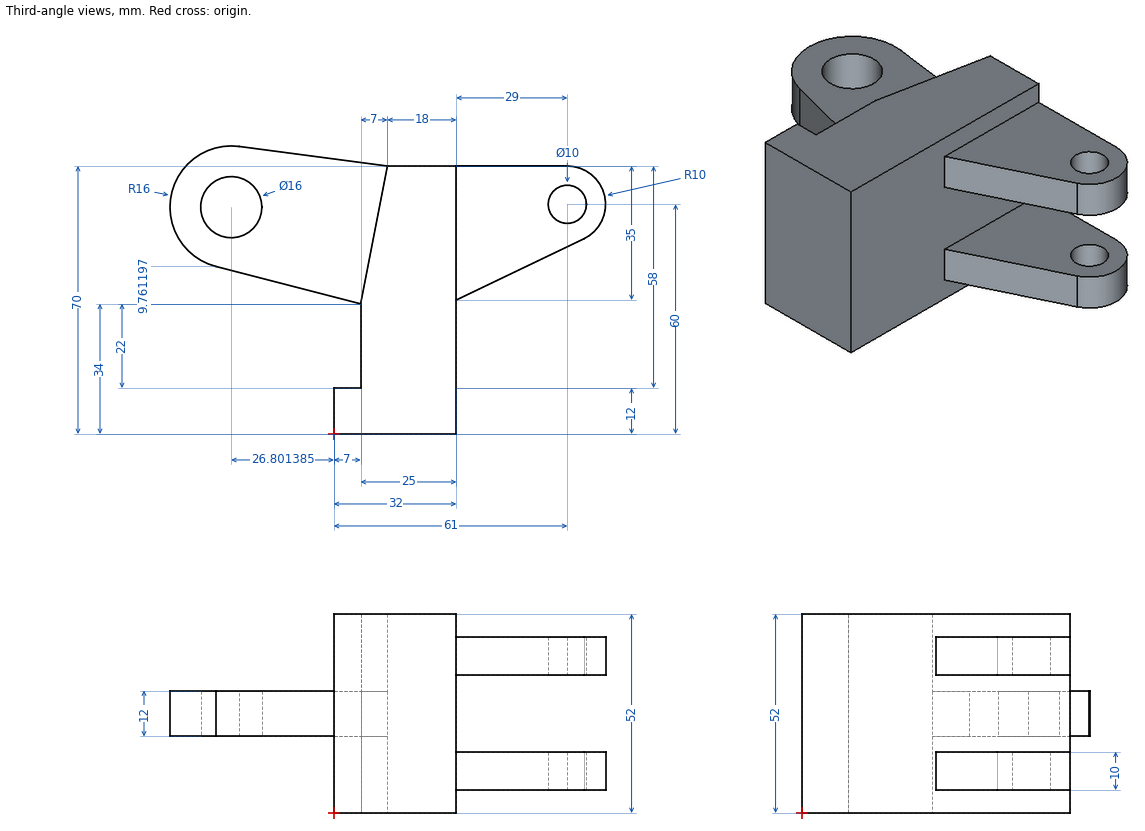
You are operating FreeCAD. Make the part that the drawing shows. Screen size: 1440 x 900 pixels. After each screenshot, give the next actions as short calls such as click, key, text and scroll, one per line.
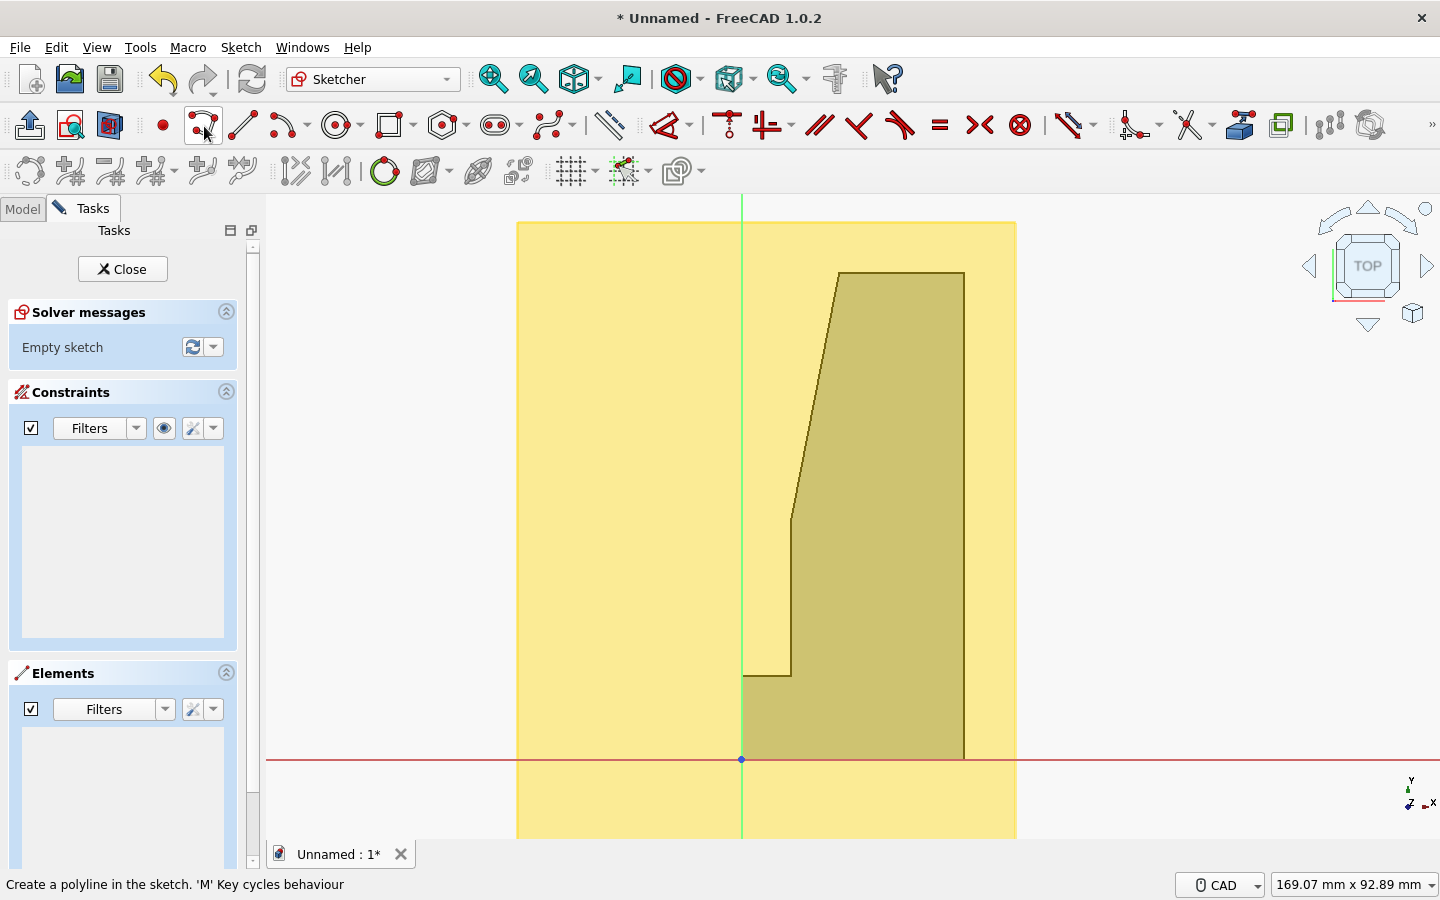
click(1165, 273)
click(964, 273)
click(964, 516)
click(1196, 406)
right_click(1196, 406)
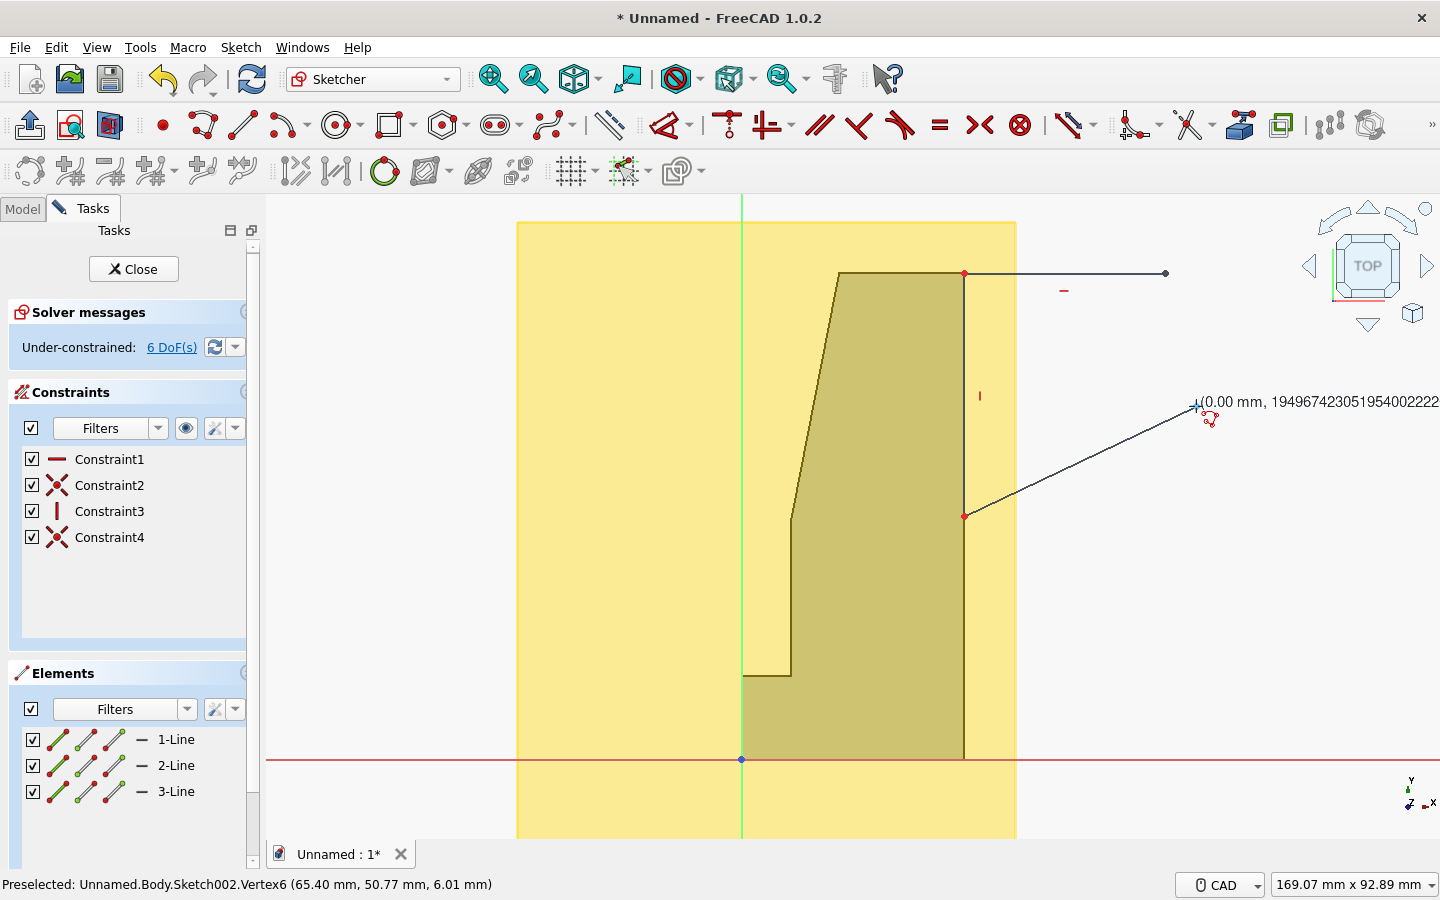
key(g)
key(3)
key(a)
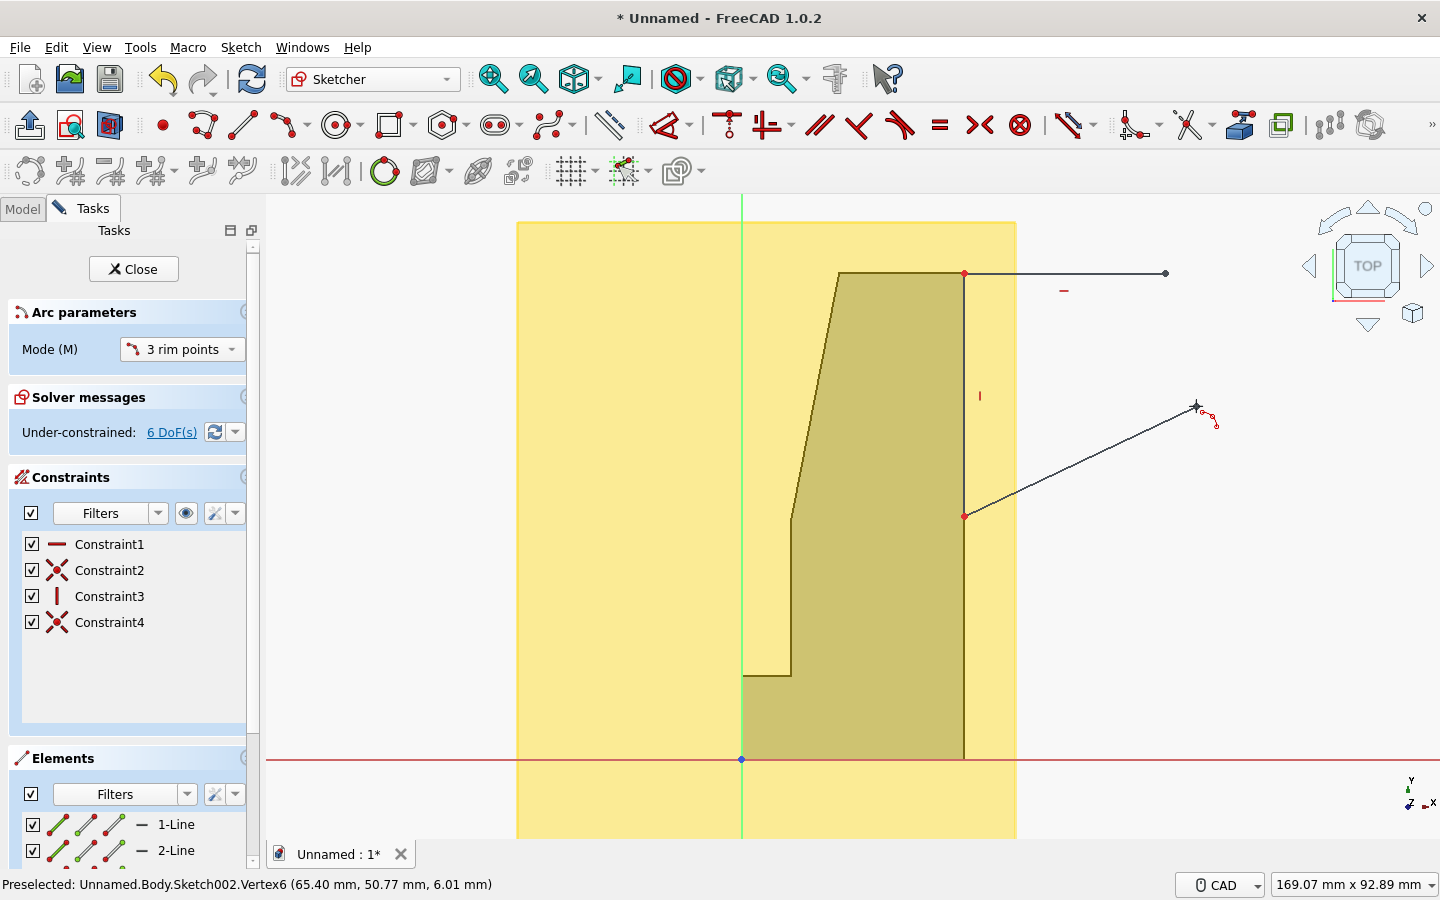
click(1196, 407)
click(1165, 274)
click(1233, 328)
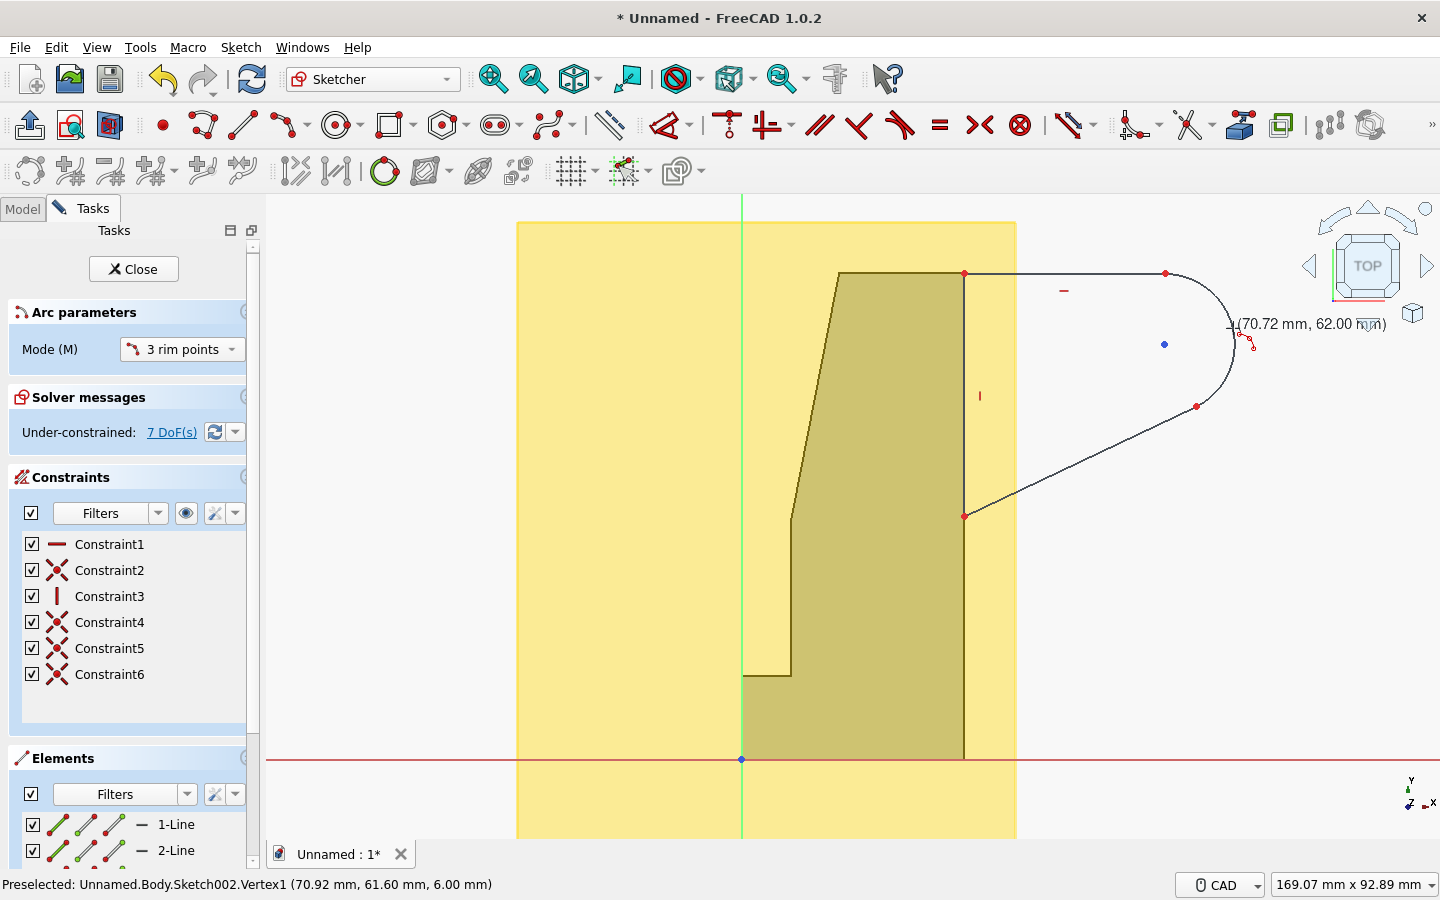
click(336, 126)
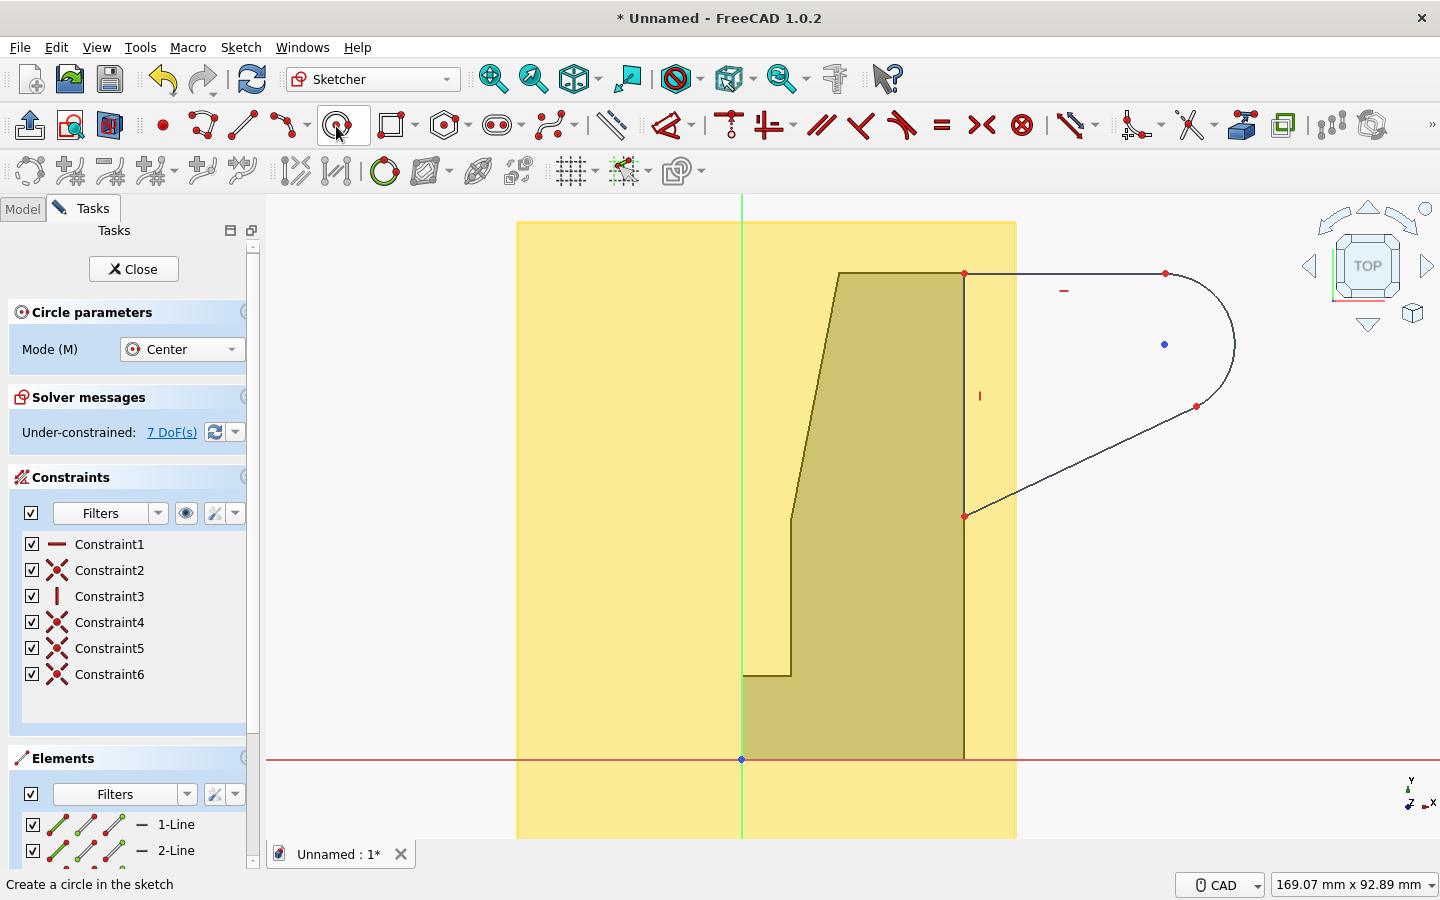
click(1165, 343)
move(1190, 318)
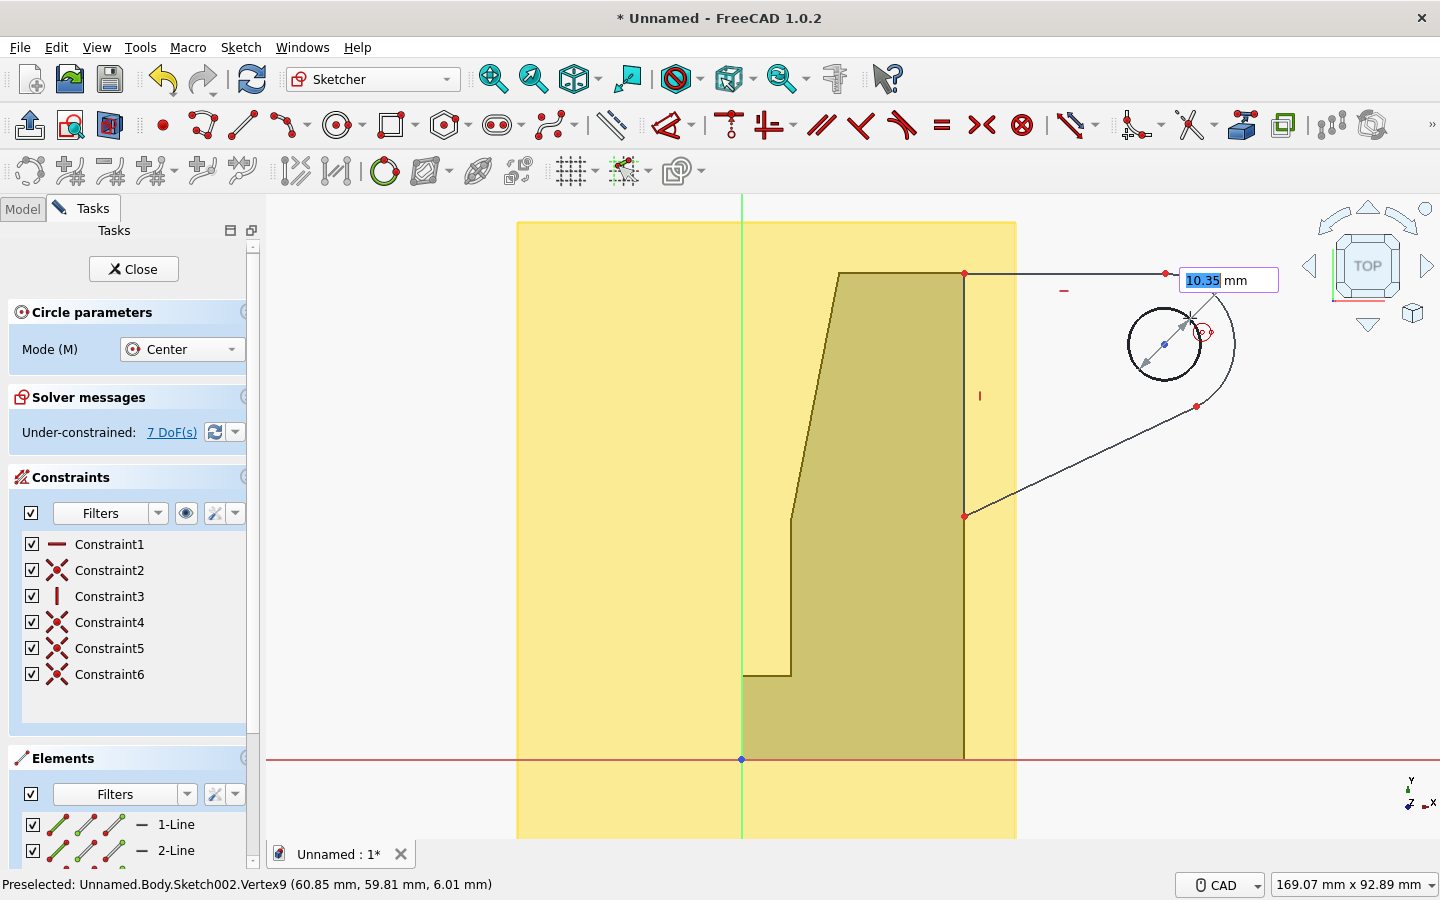
text(10)
key(Return)
key(Escape)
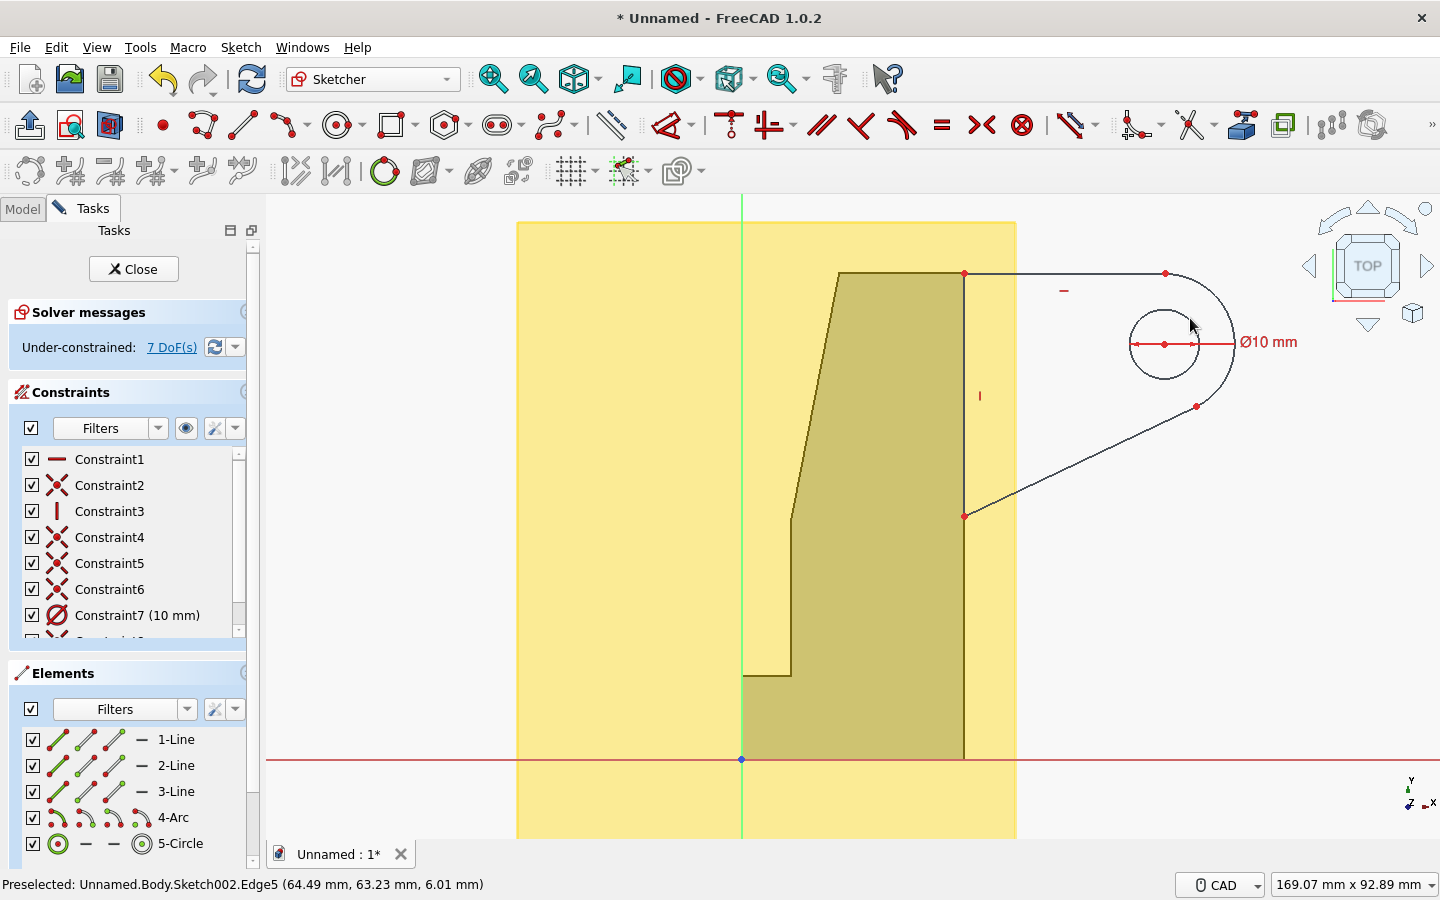
click(1105, 274)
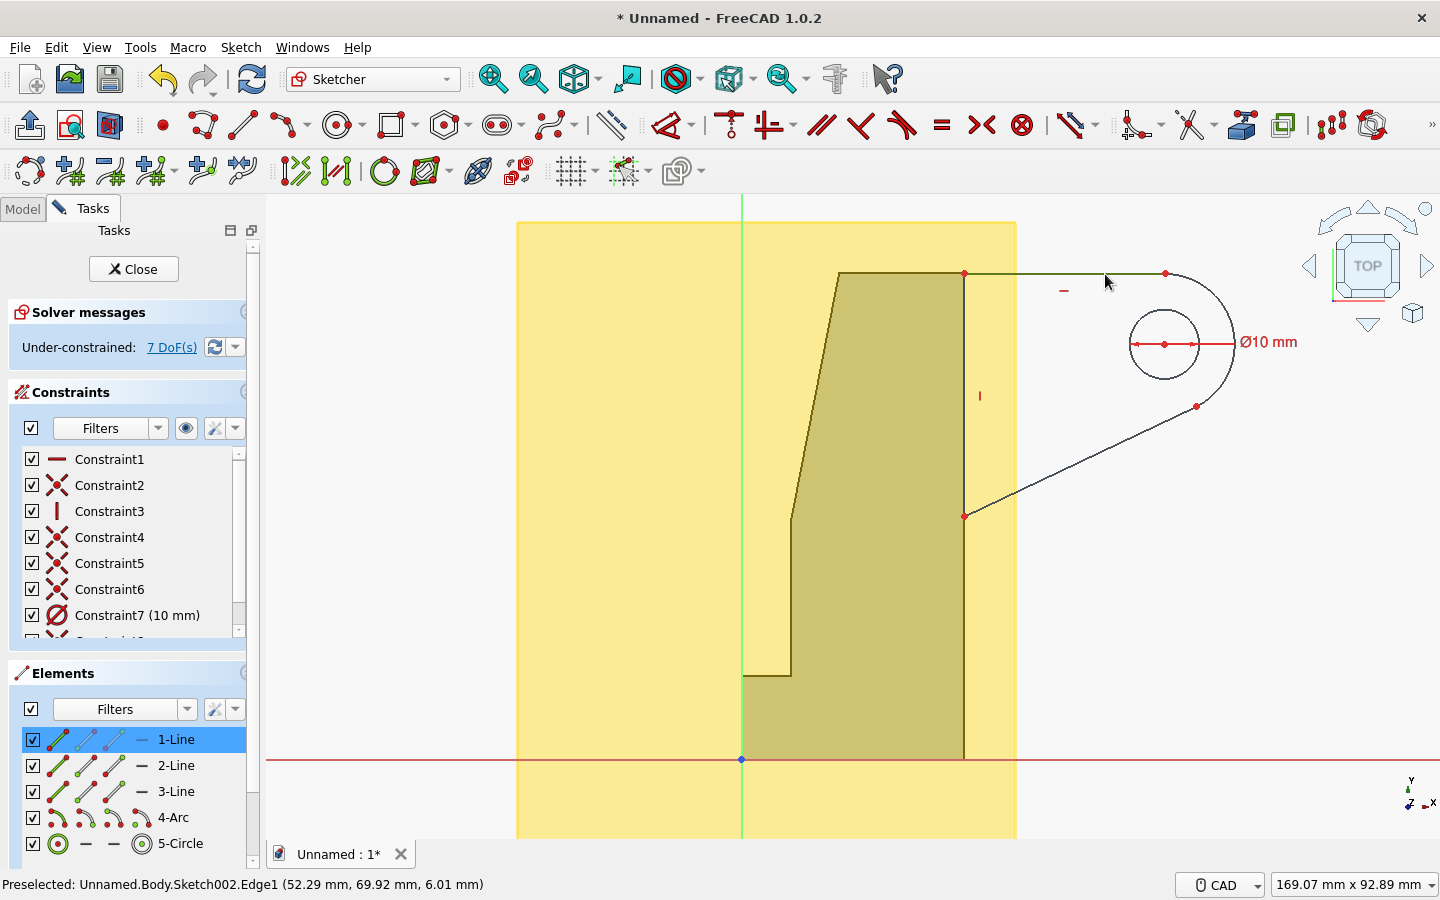
click(1231, 365)